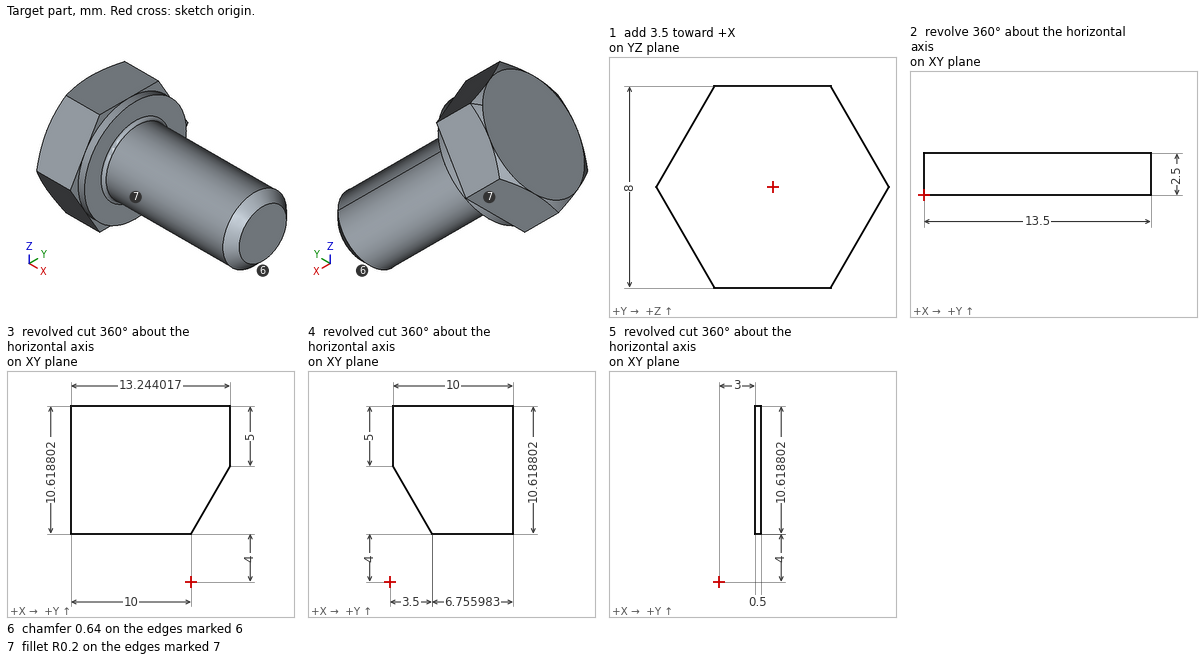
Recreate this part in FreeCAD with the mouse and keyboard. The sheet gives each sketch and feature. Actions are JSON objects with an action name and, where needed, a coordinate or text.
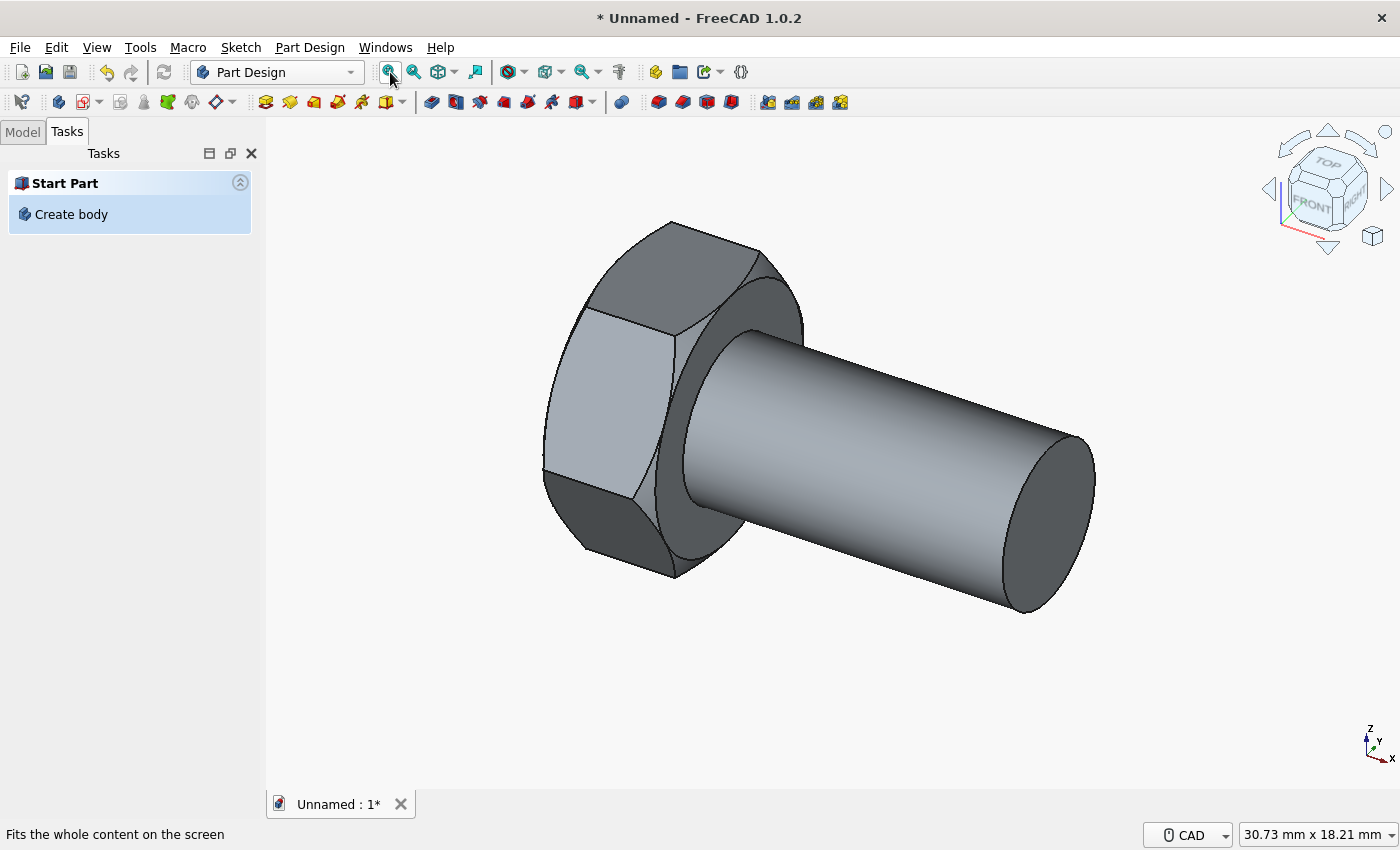
{"action": "left_click", "coordinate": [84, 102]}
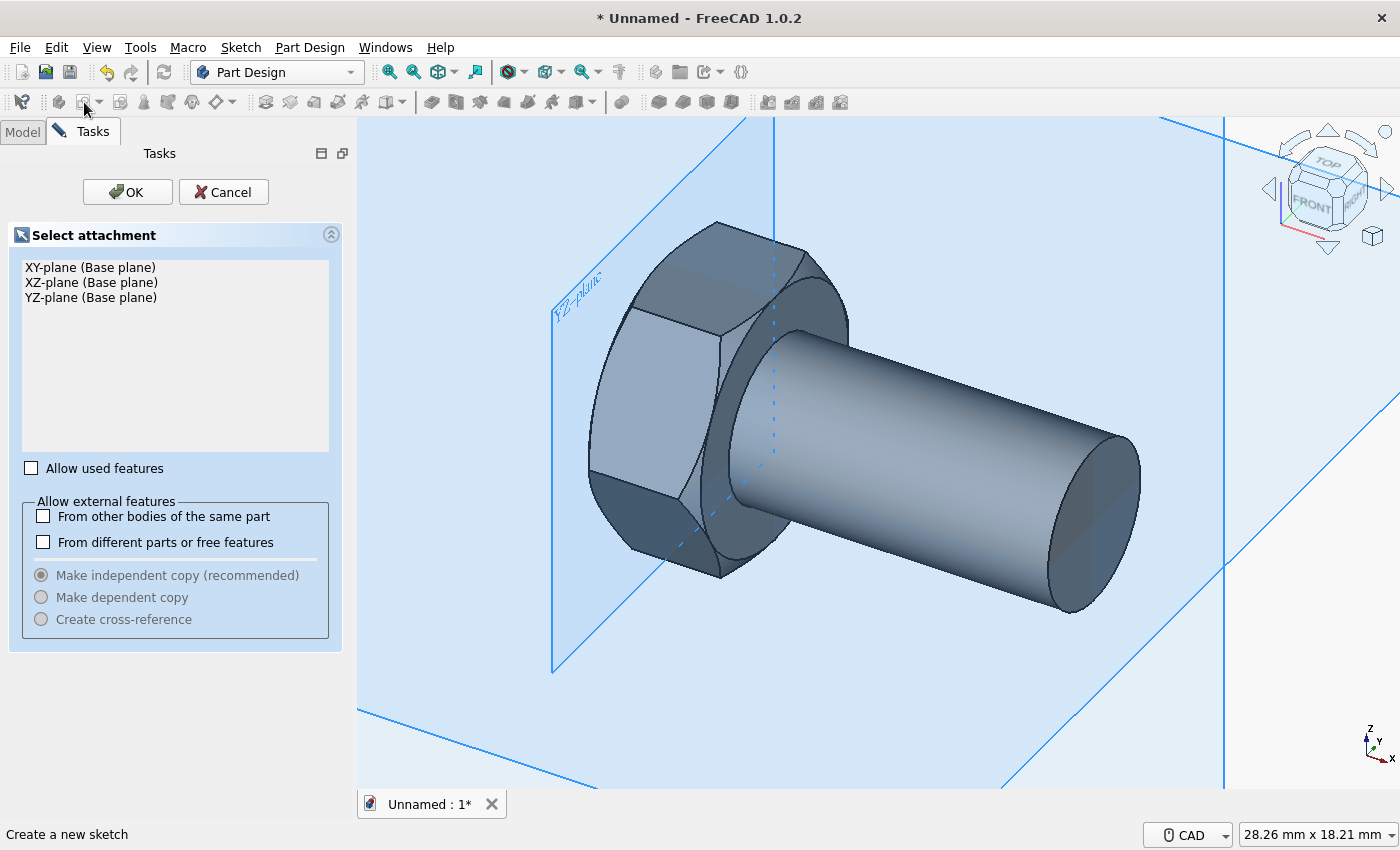
{"action": "left_click", "coordinate": [82, 268]}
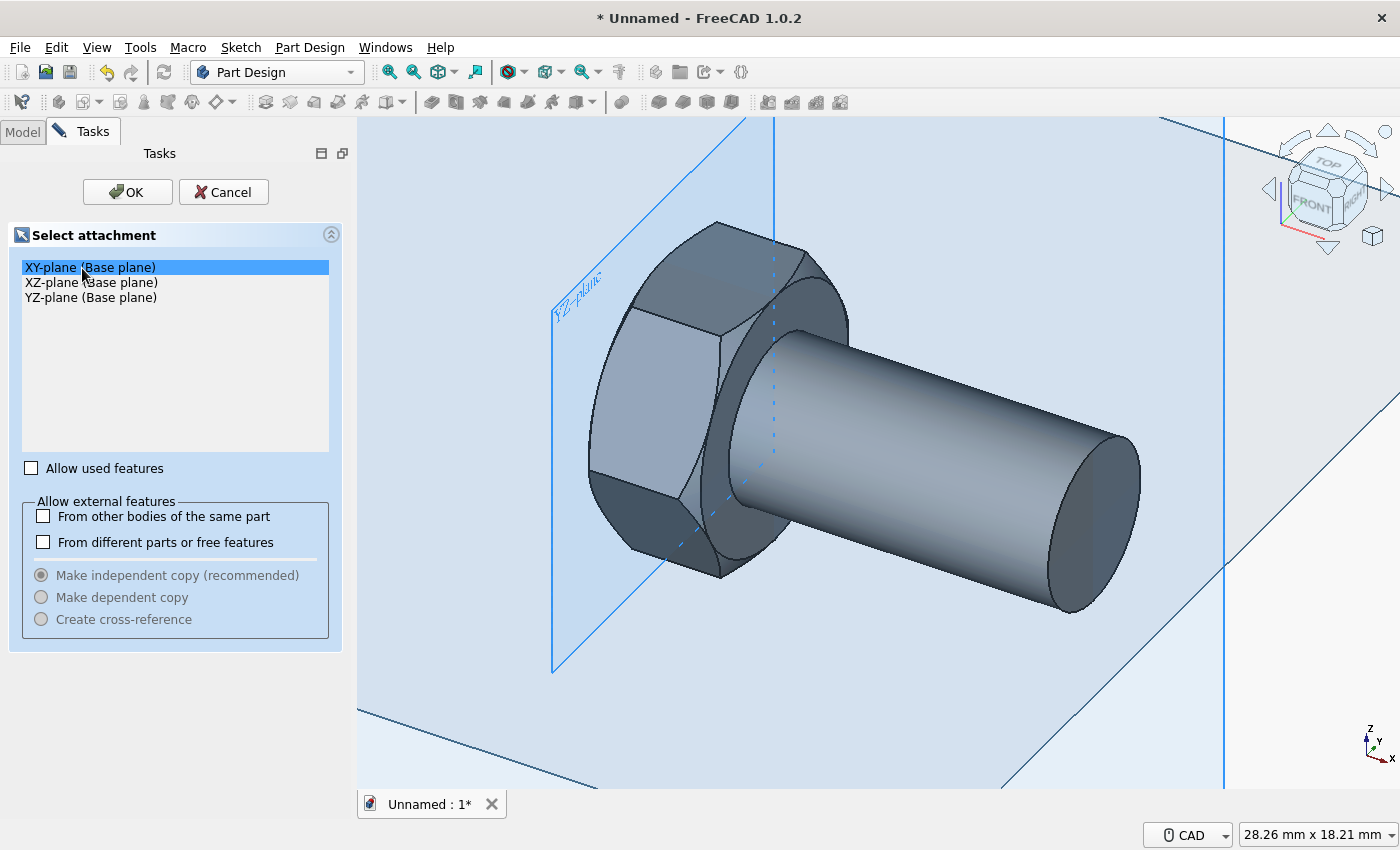
{"action": "left_click", "coordinate": [128, 192]}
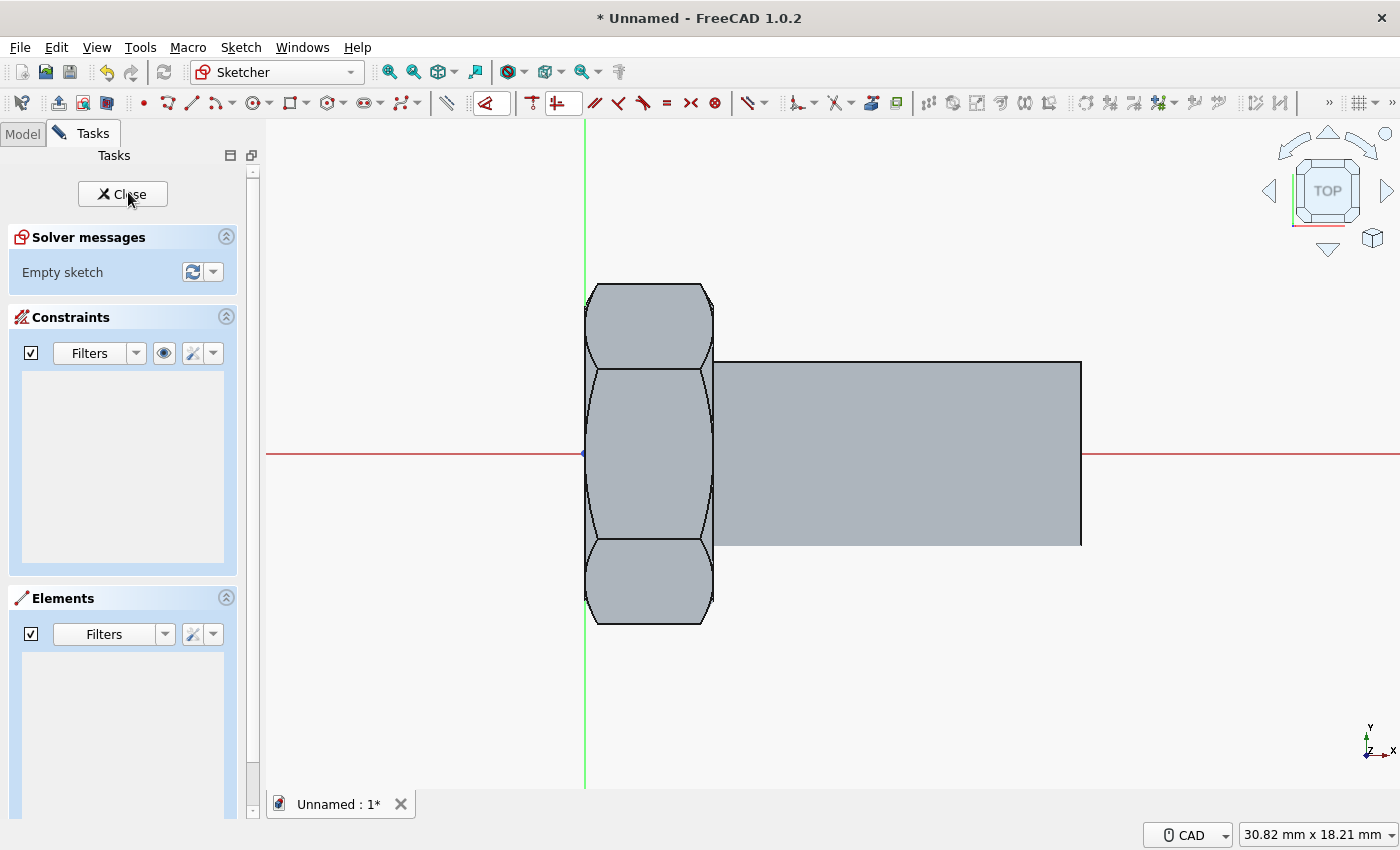
{"action": "left_click", "coordinate": [108, 104]}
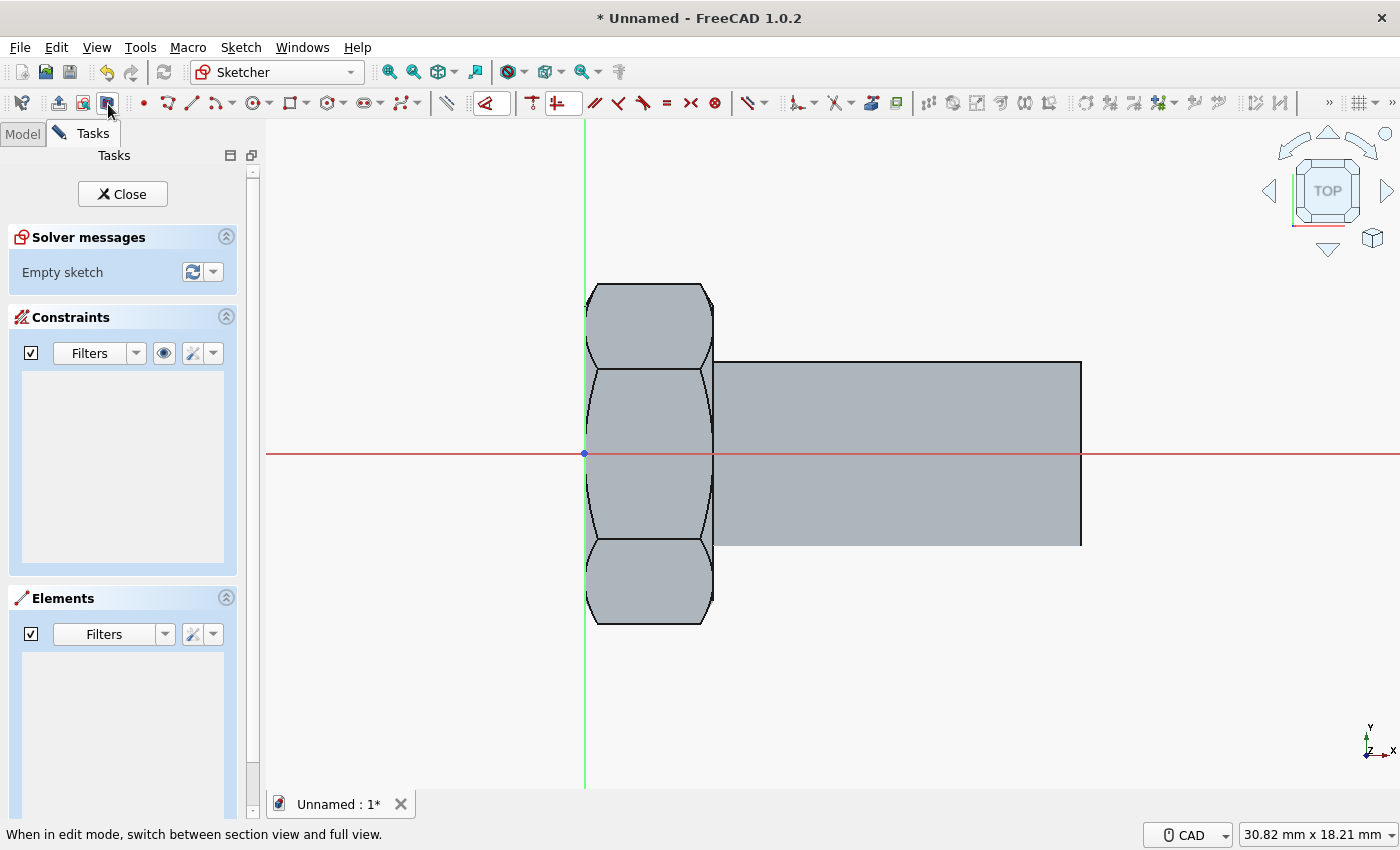
{"action": "scroll", "coordinate": [999, 761], "scroll_direction": "down", "scroll_amount": 2}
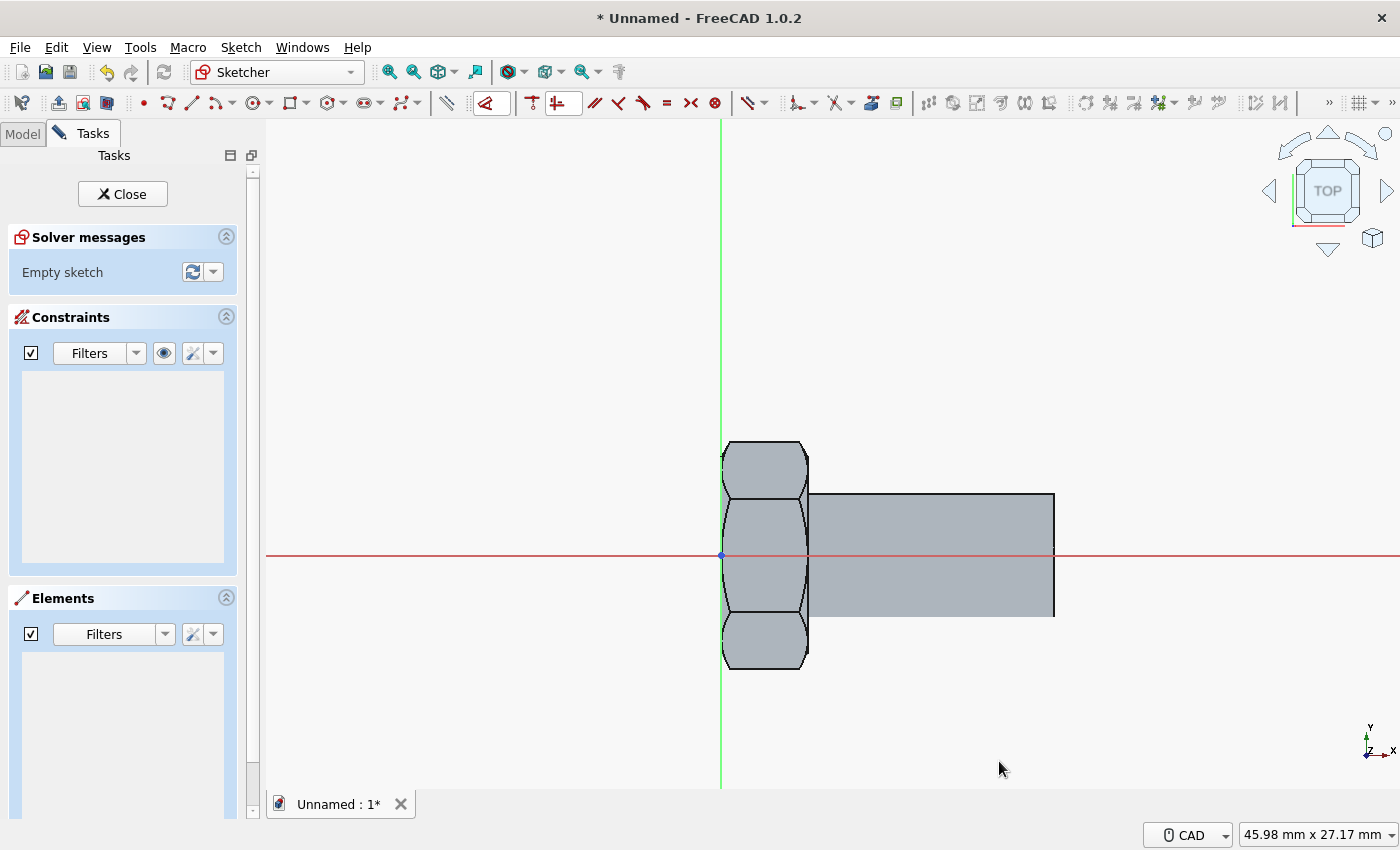
{"action": "left_click", "coordinate": [290, 104]}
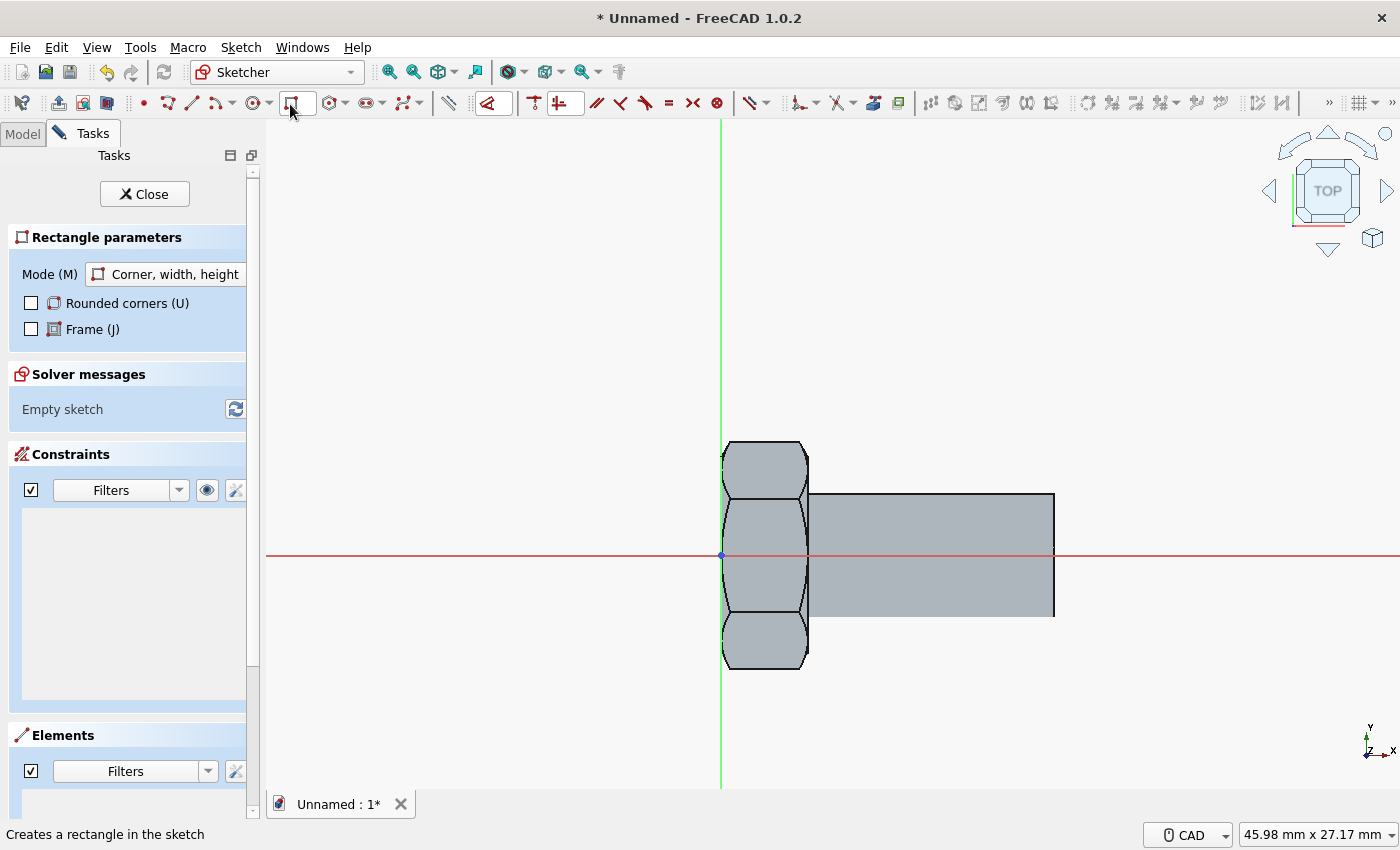
{"action": "scroll", "coordinate": [795, 195], "scroll_direction": "up", "scroll_amount": 2}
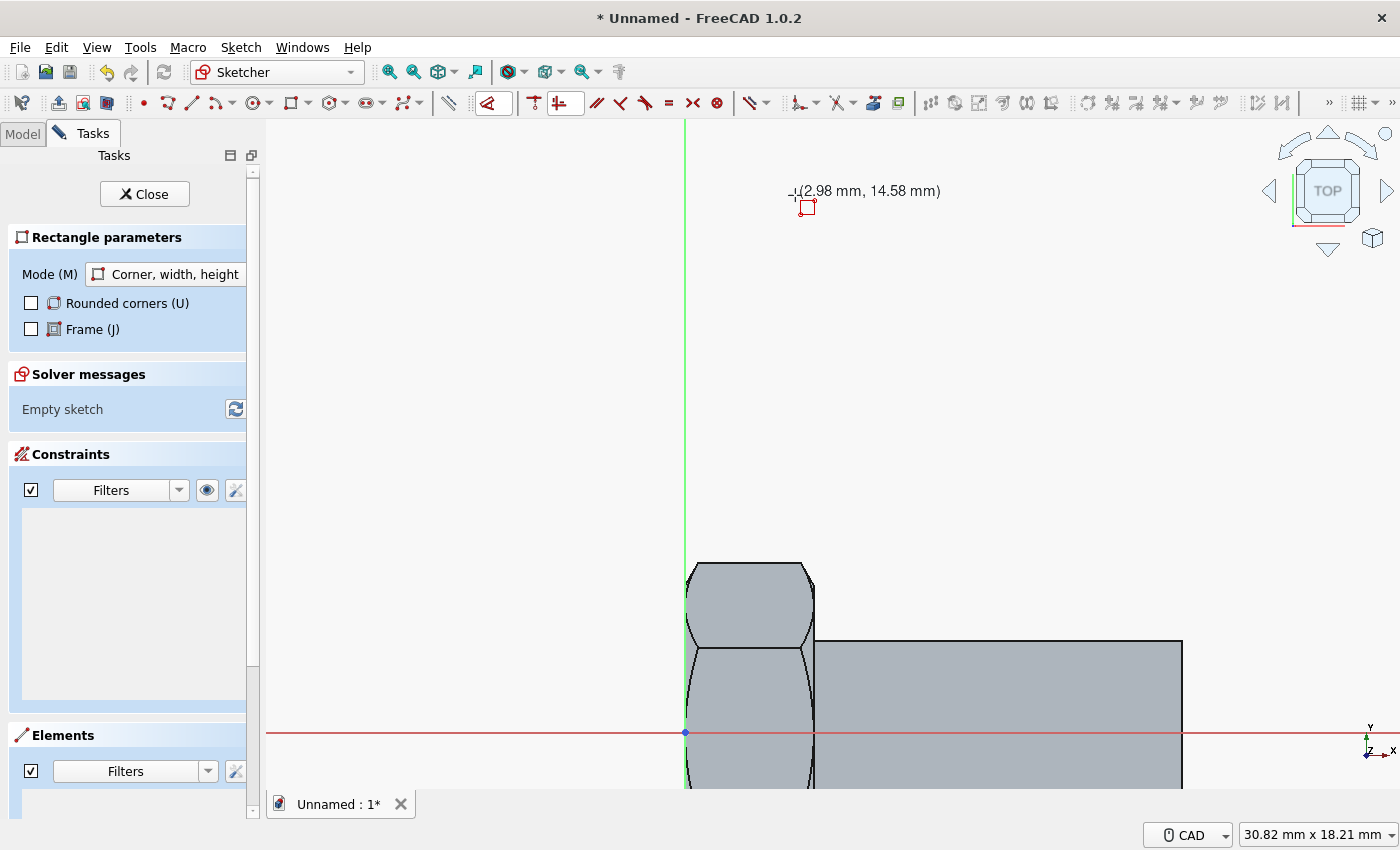
{"action": "left_click", "coordinate": [795, 195]}
{"action": "mouse_move", "coordinate": [814, 586]}